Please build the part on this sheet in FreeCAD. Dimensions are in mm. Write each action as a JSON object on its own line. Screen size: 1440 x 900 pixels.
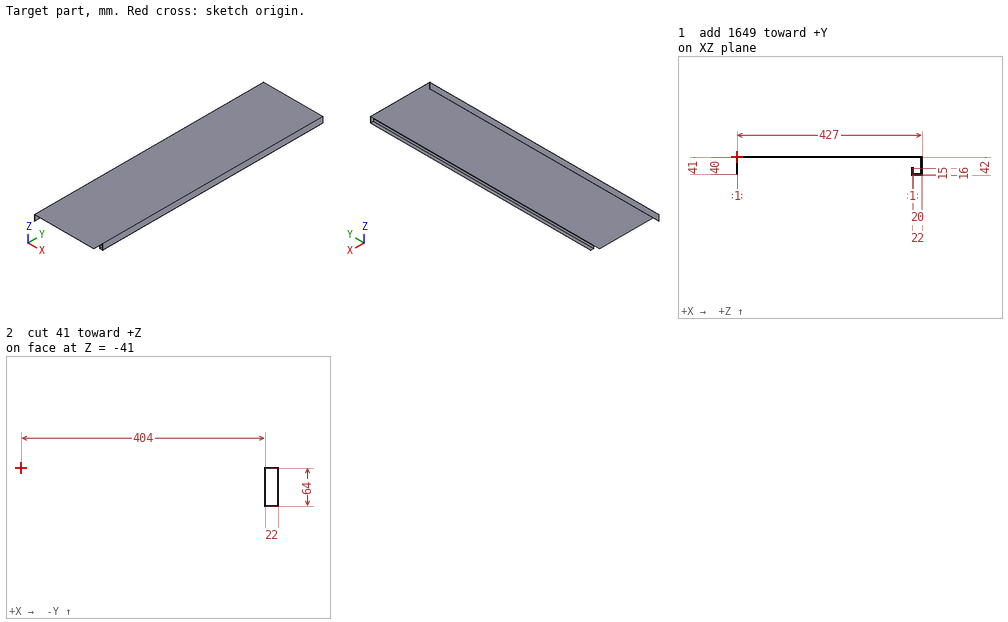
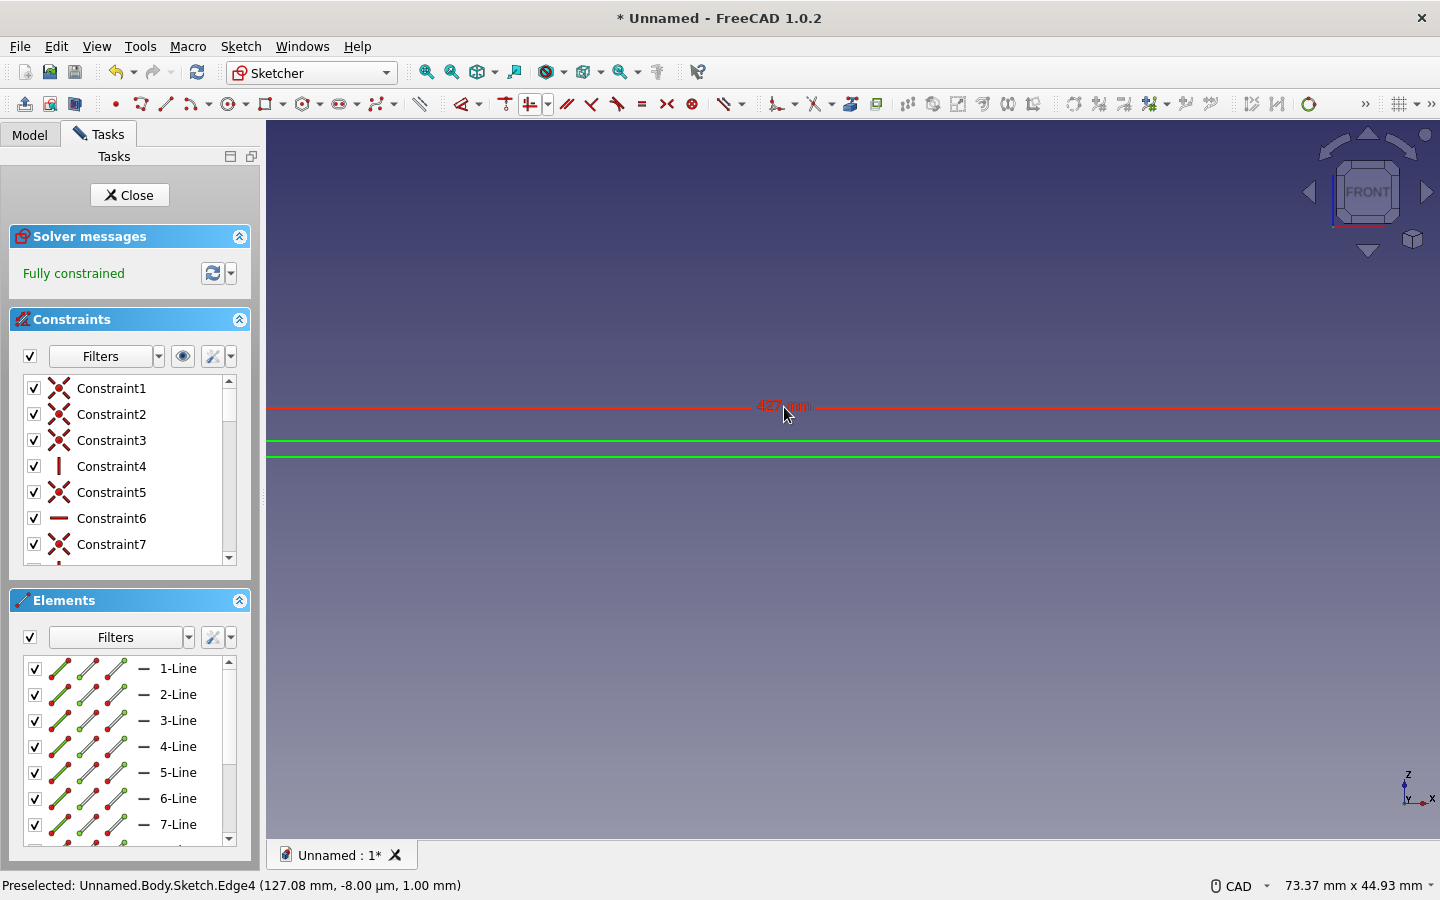
{"action": "left_click", "coordinate": [130, 195]}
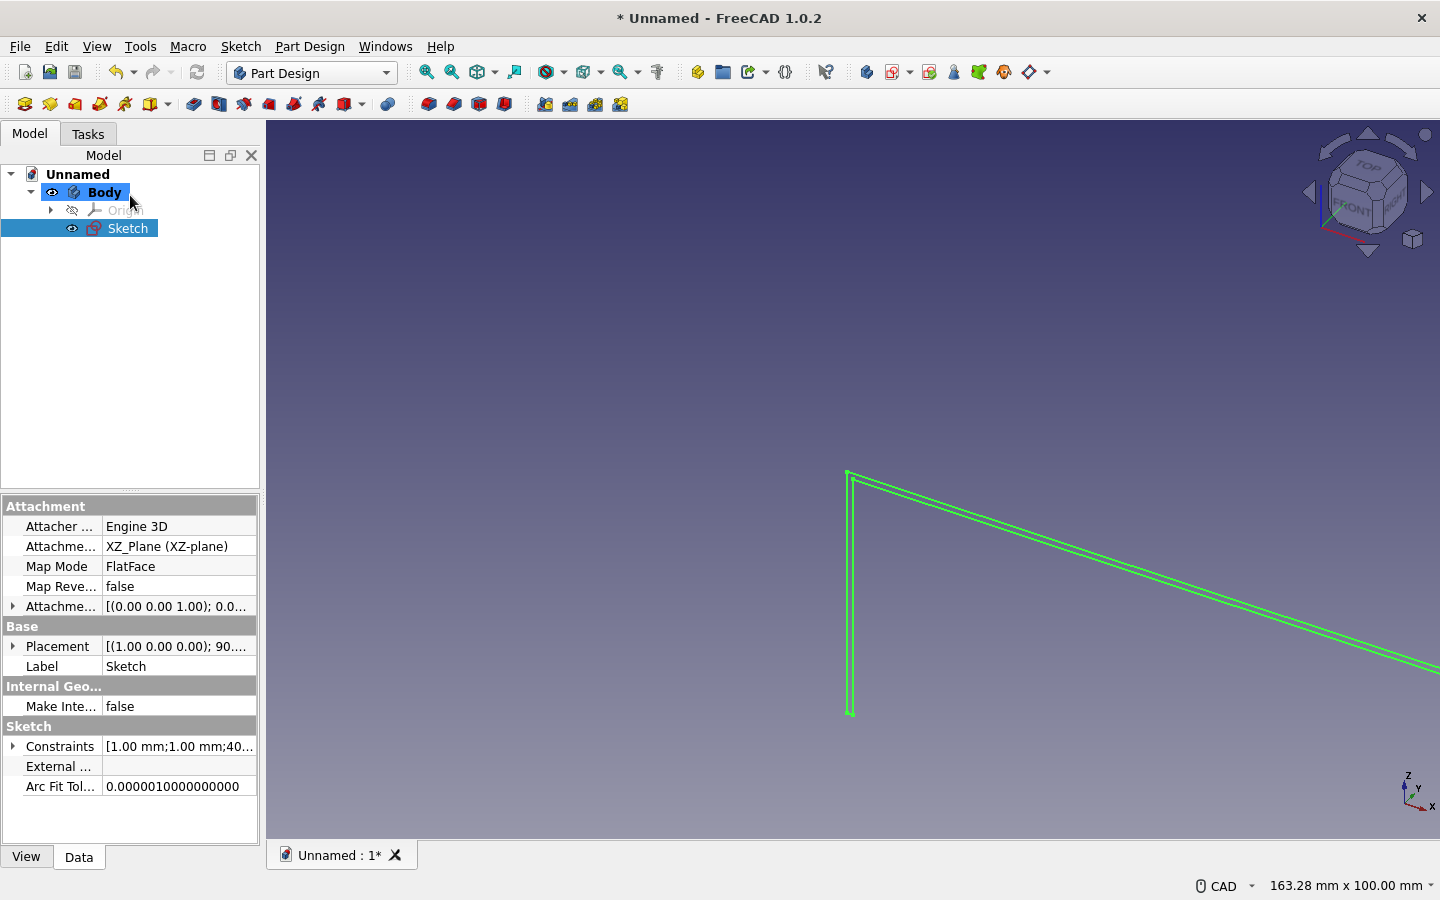
{"action": "left_click", "coordinate": [25, 104]}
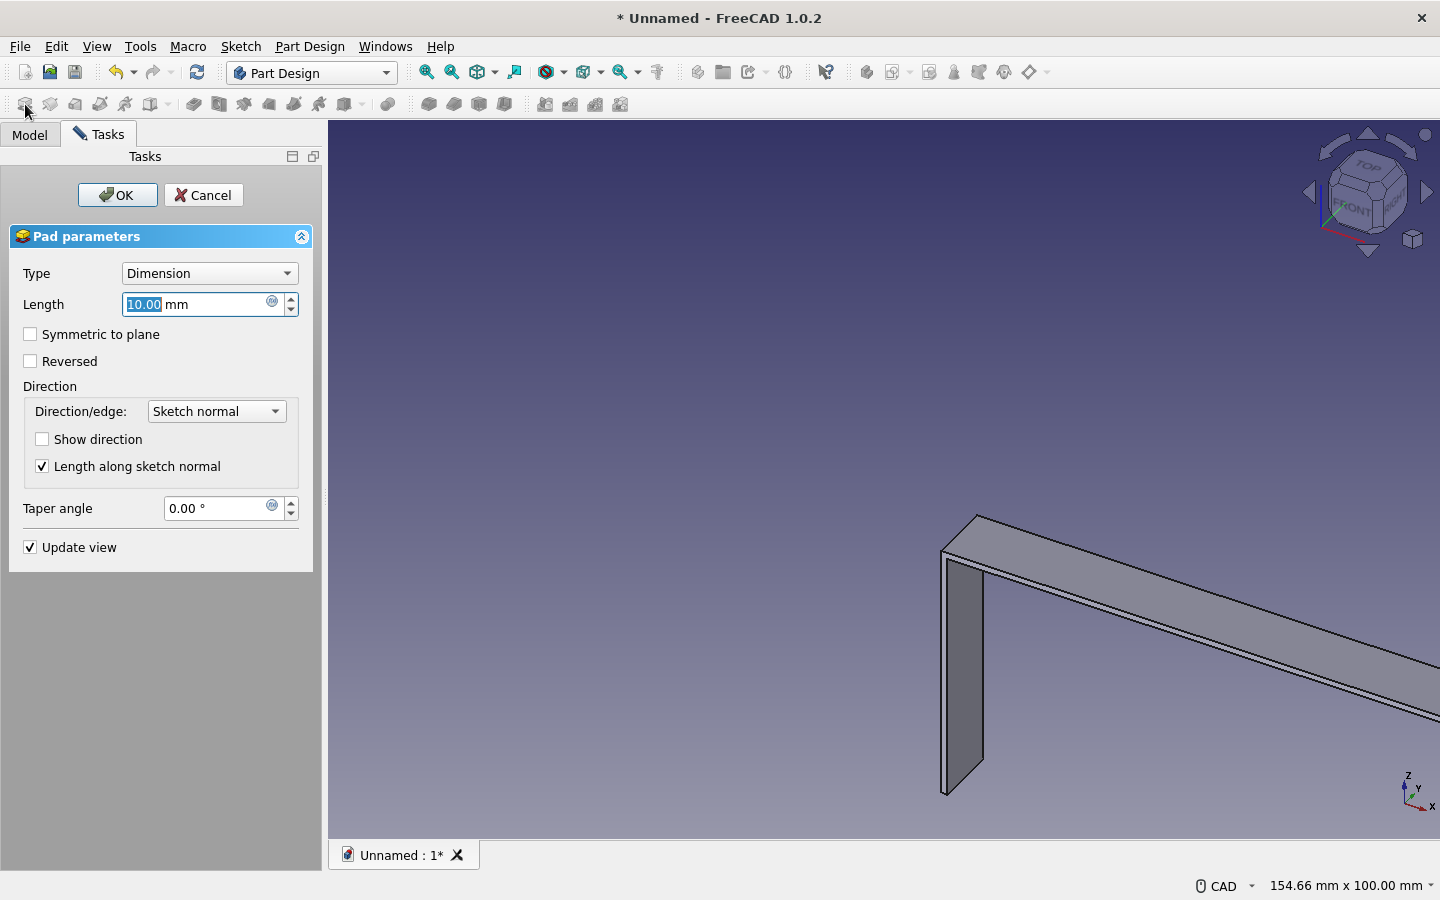
{"action": "type", "text": "1649"}
{"action": "key", "text": "Tab"}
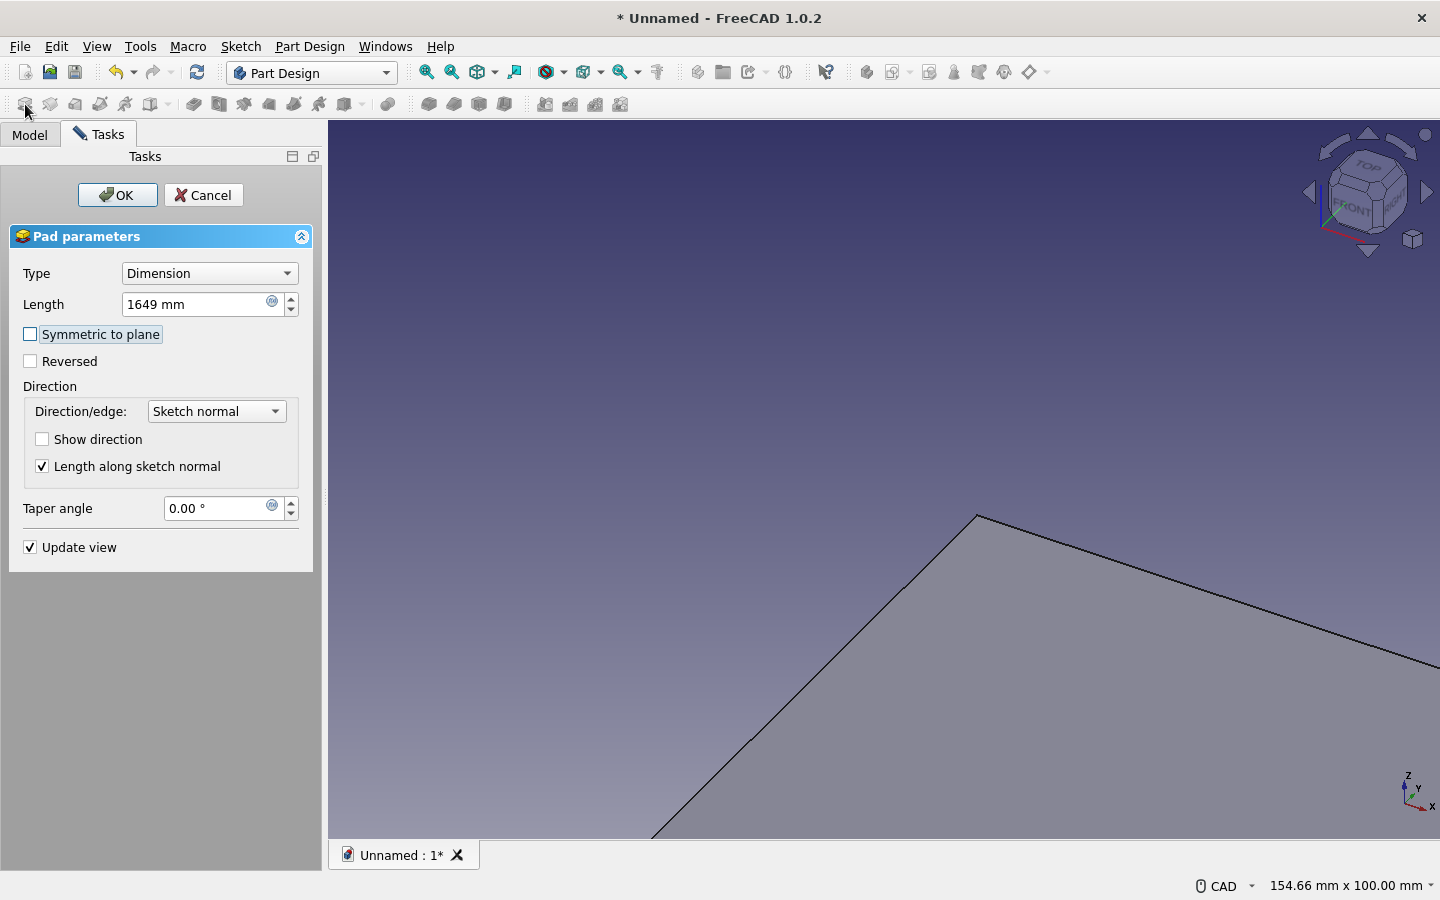
{"action": "left_click", "coordinate": [31, 361]}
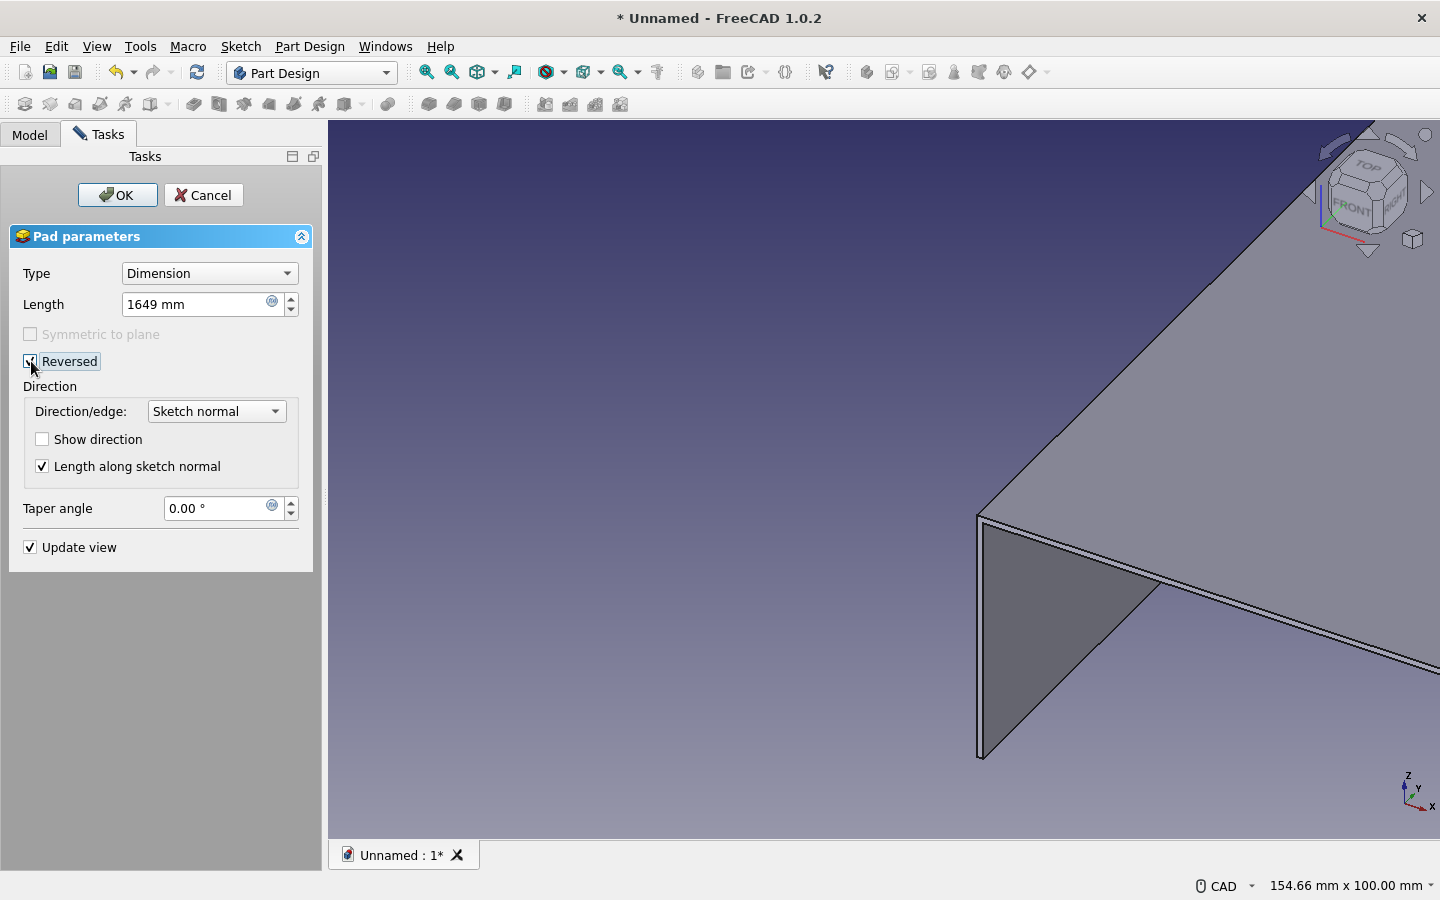
{"action": "left_click", "coordinate": [118, 195]}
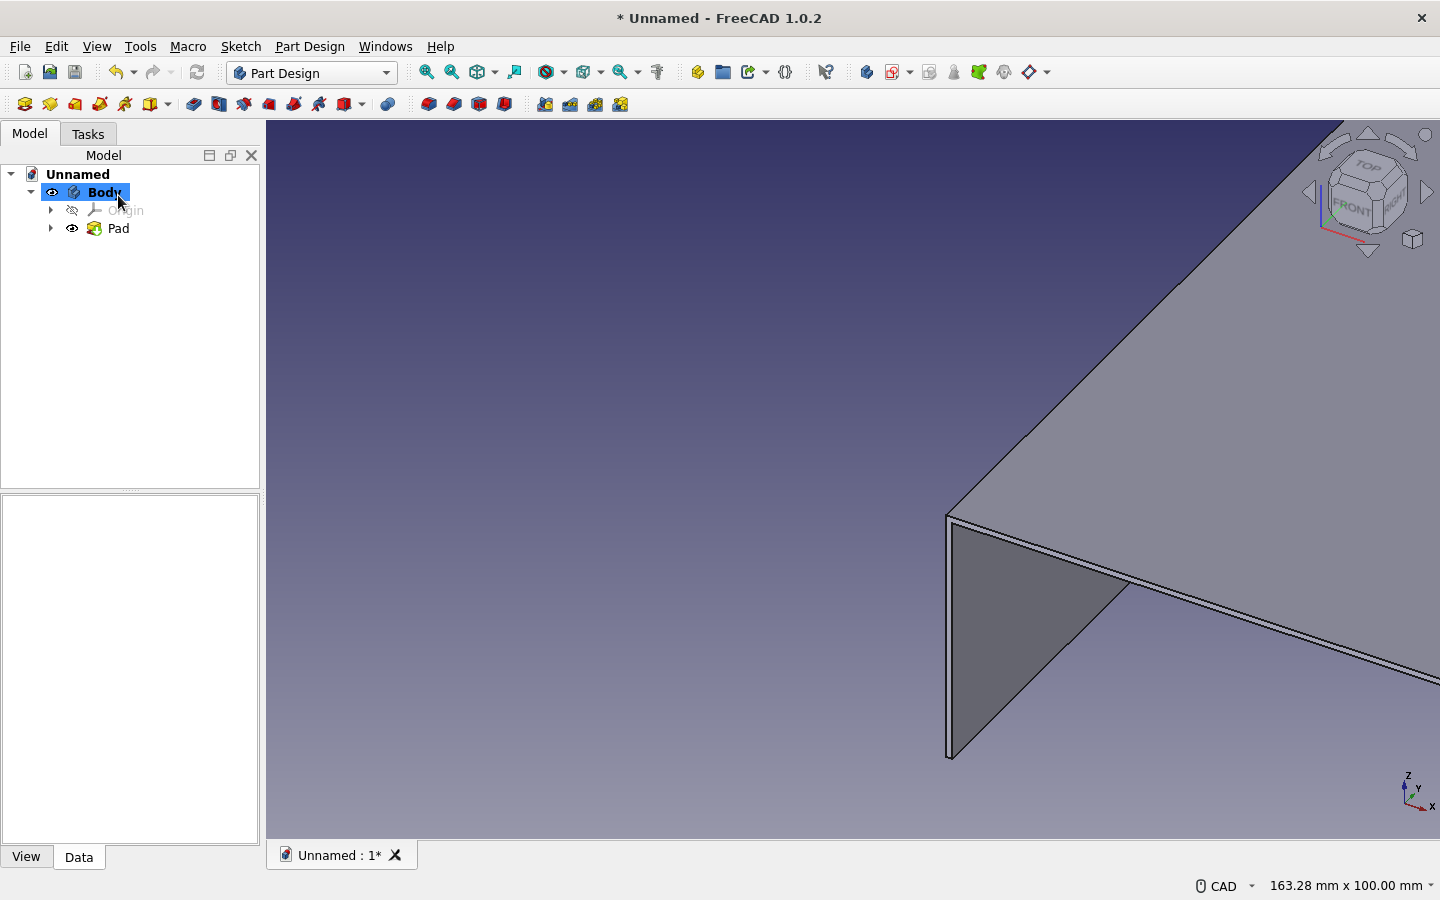
{"action": "left_click", "coordinate": [427, 72]}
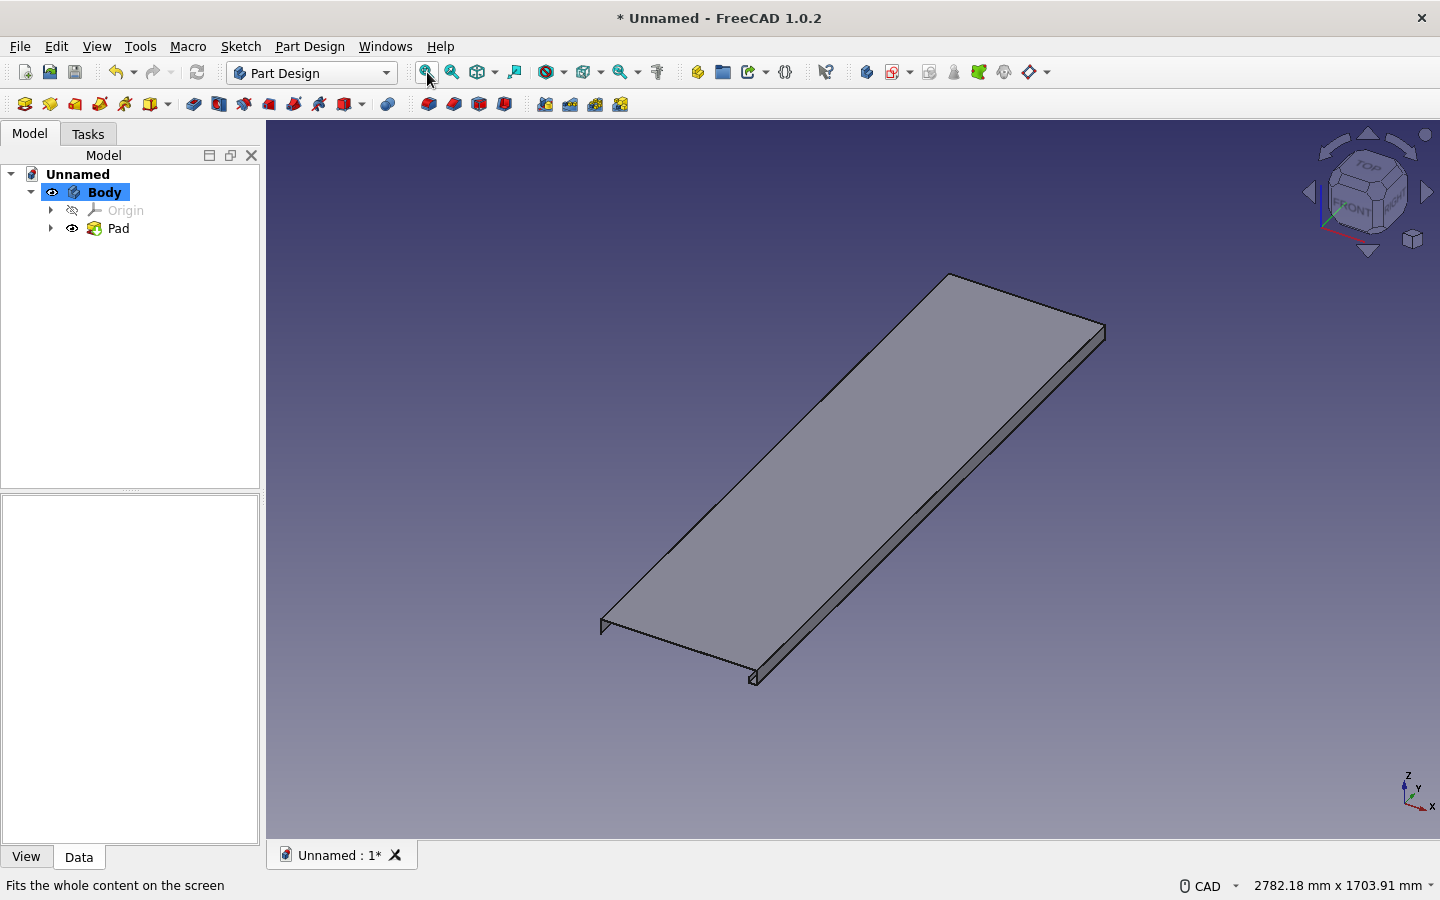
{"action": "key", "text": "5"}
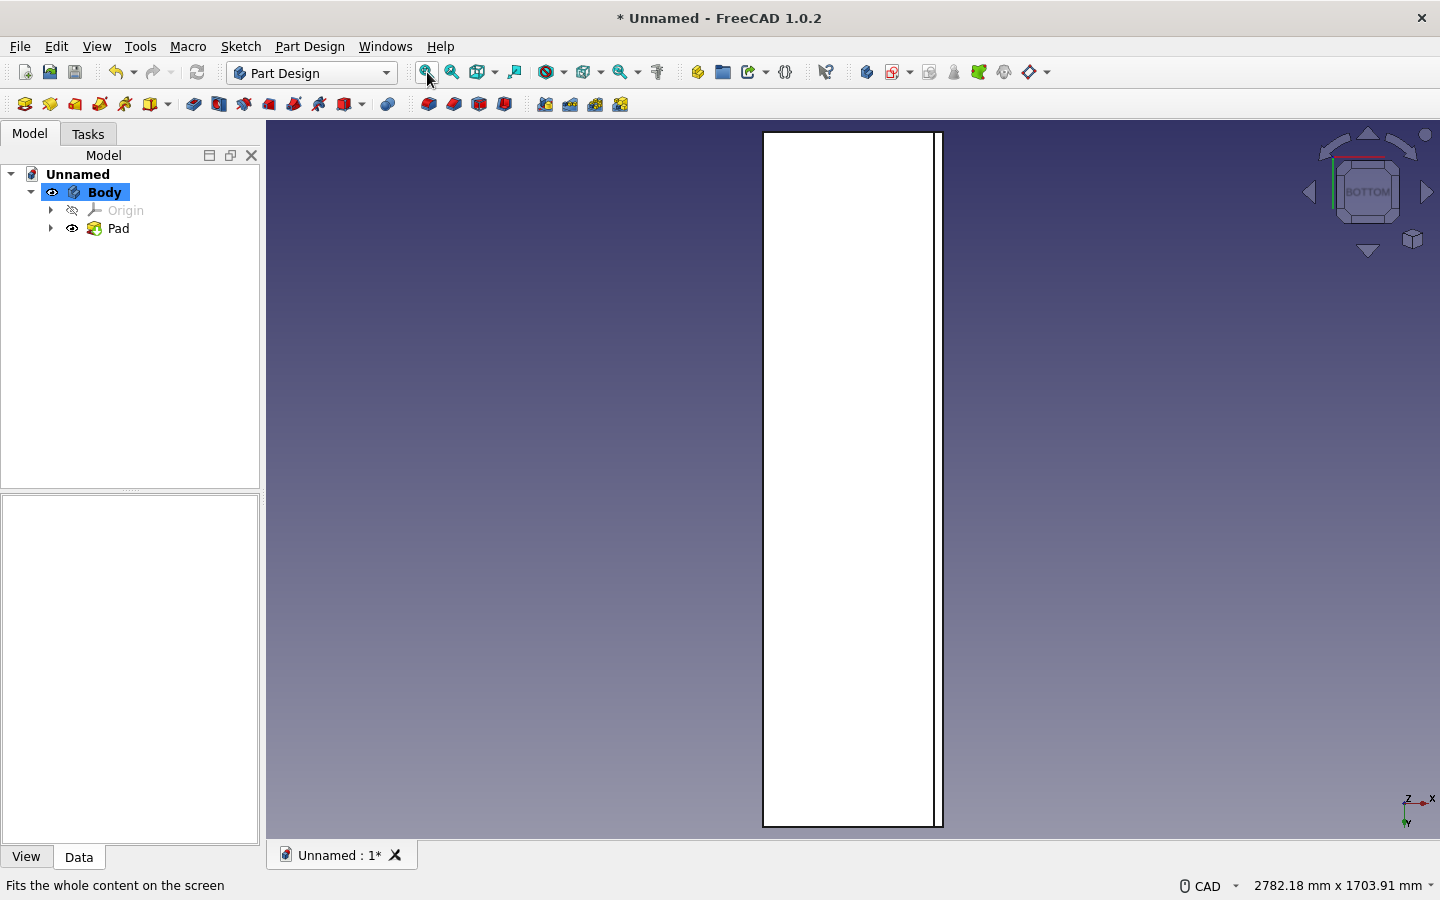
{"action": "scroll", "coordinate": [938, 777], "scroll_direction": "up", "scroll_amount": 5}